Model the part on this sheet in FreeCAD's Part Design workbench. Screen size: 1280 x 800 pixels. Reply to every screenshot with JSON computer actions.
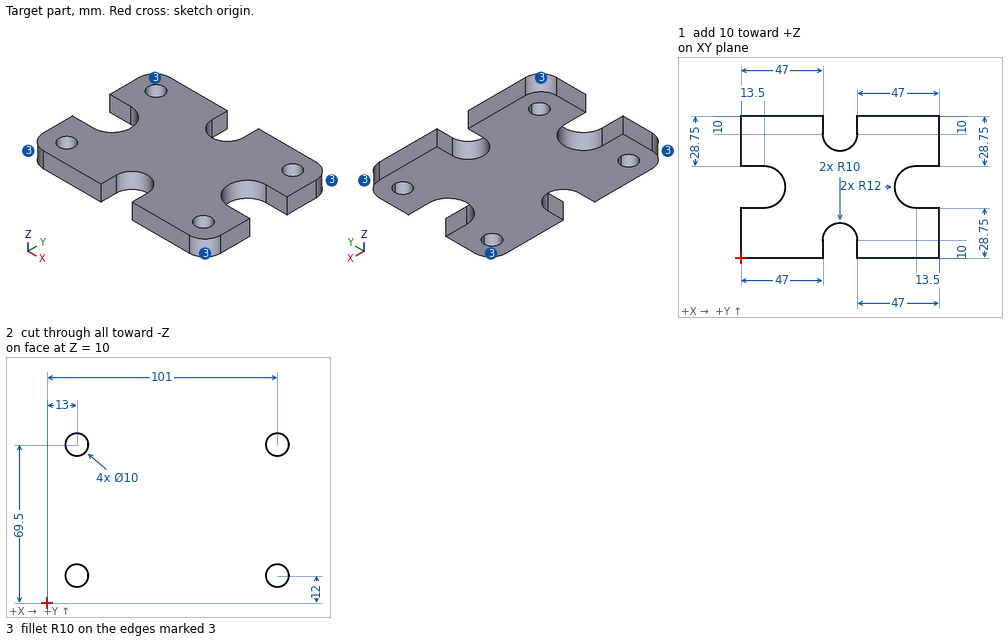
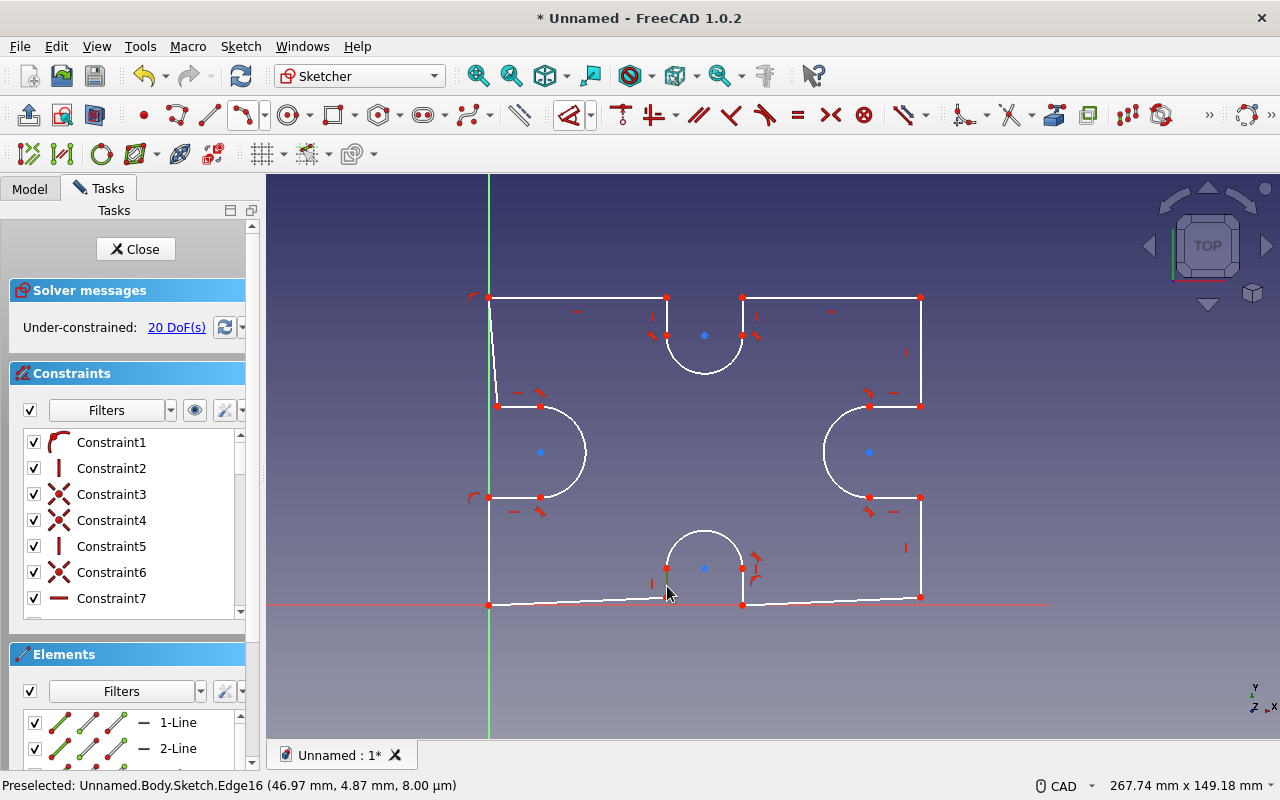
{"action": "left_click", "coordinate": [727, 538]}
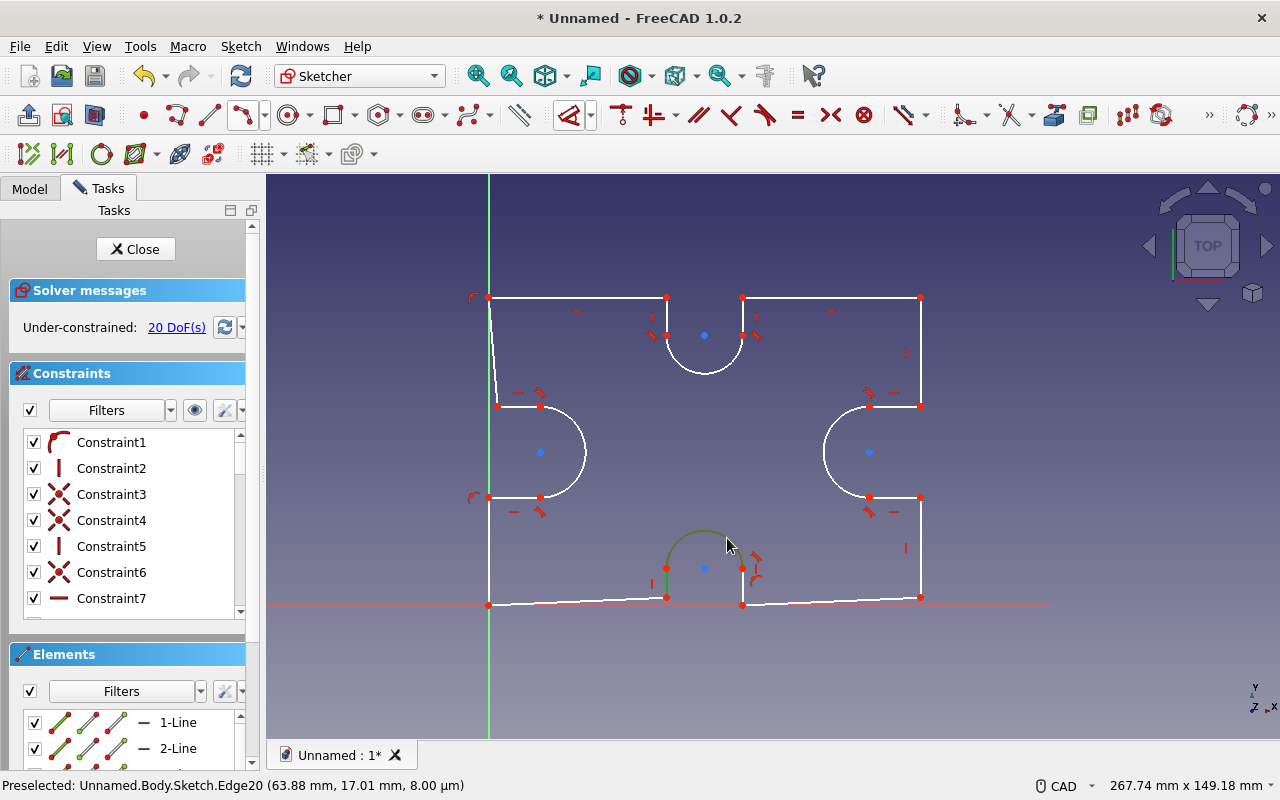
{"action": "left_click", "coordinate": [765, 116]}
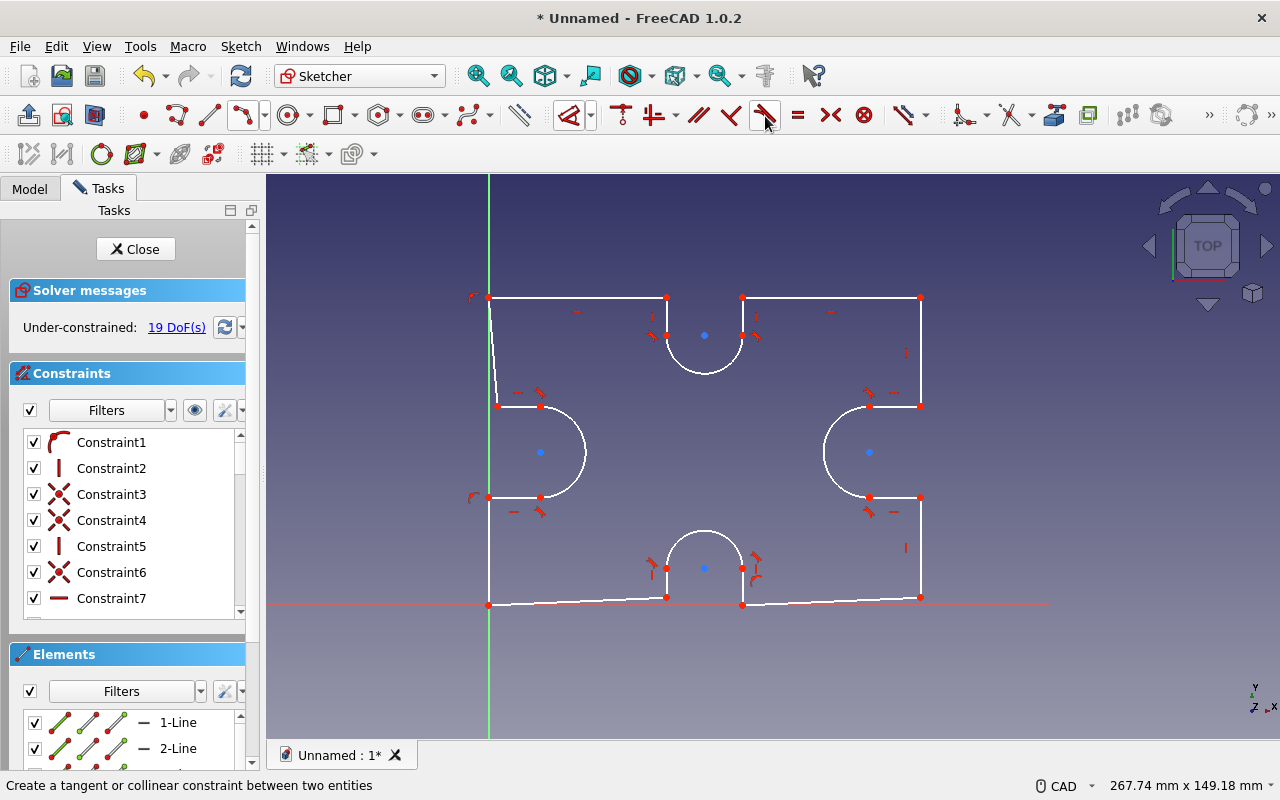
{"action": "left_click", "coordinate": [796, 603]}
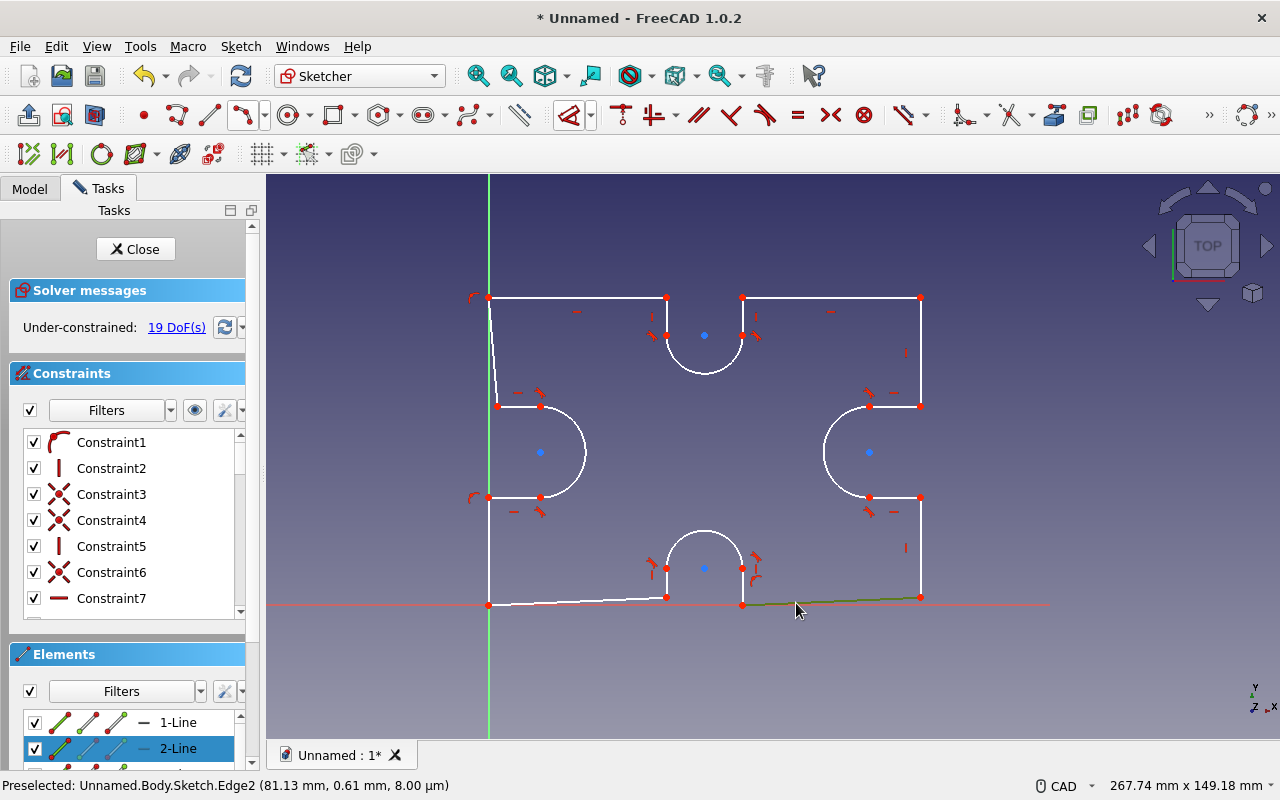
{"action": "left_click", "coordinate": [676, 116]}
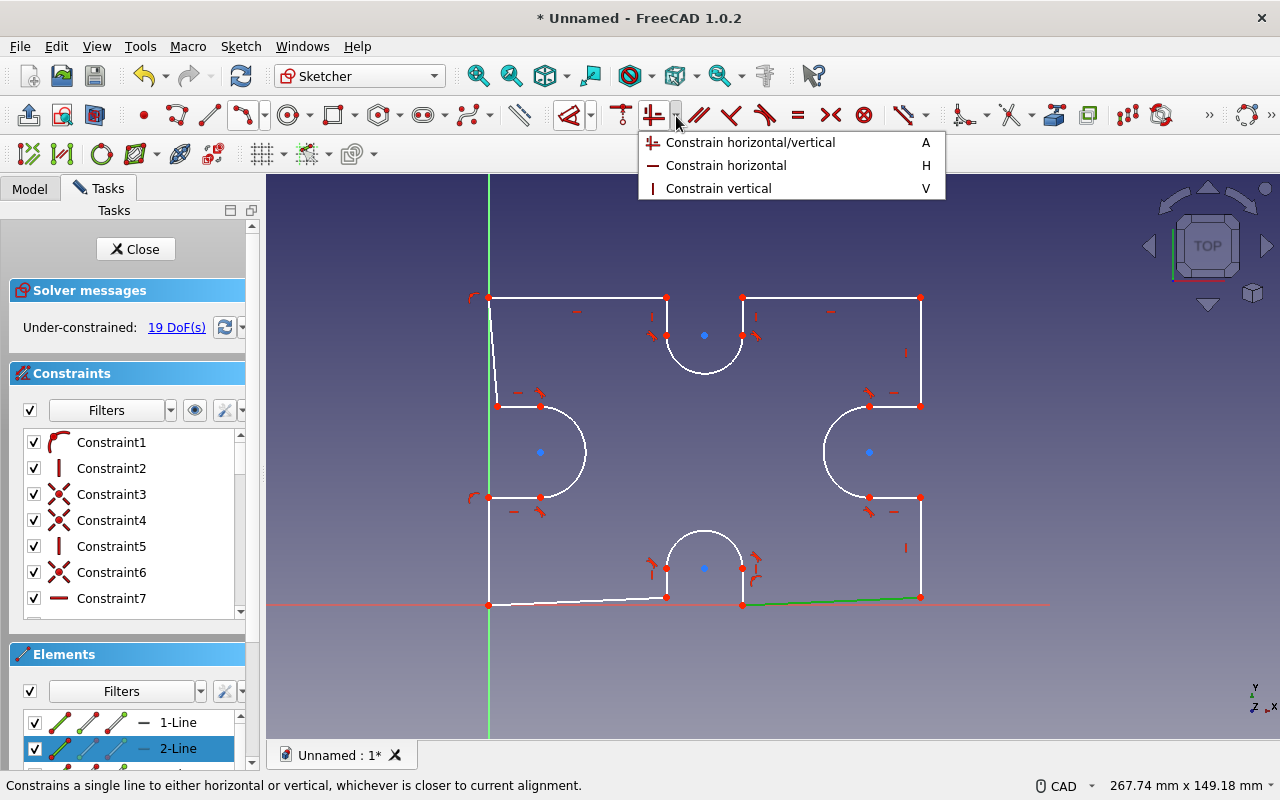
{"action": "left_click", "coordinate": [792, 166]}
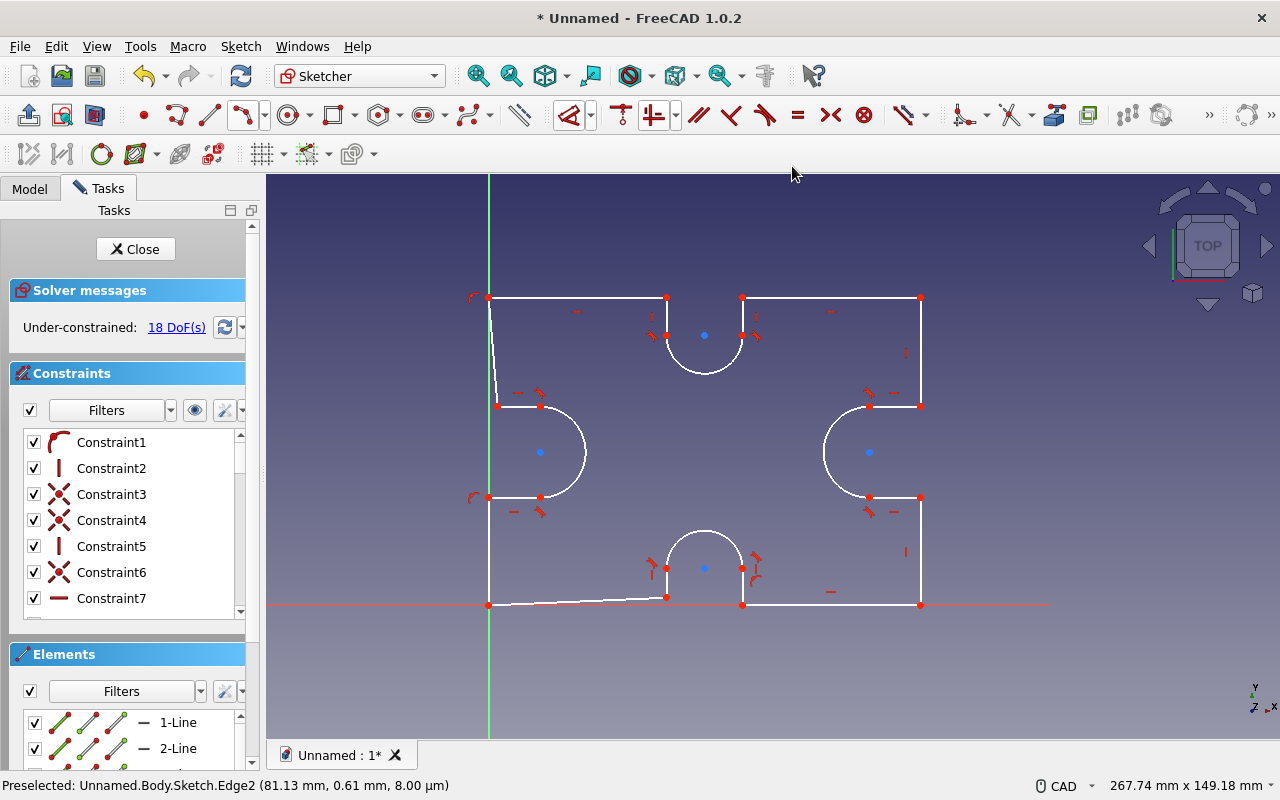
{"action": "left_click", "coordinate": [491, 330]}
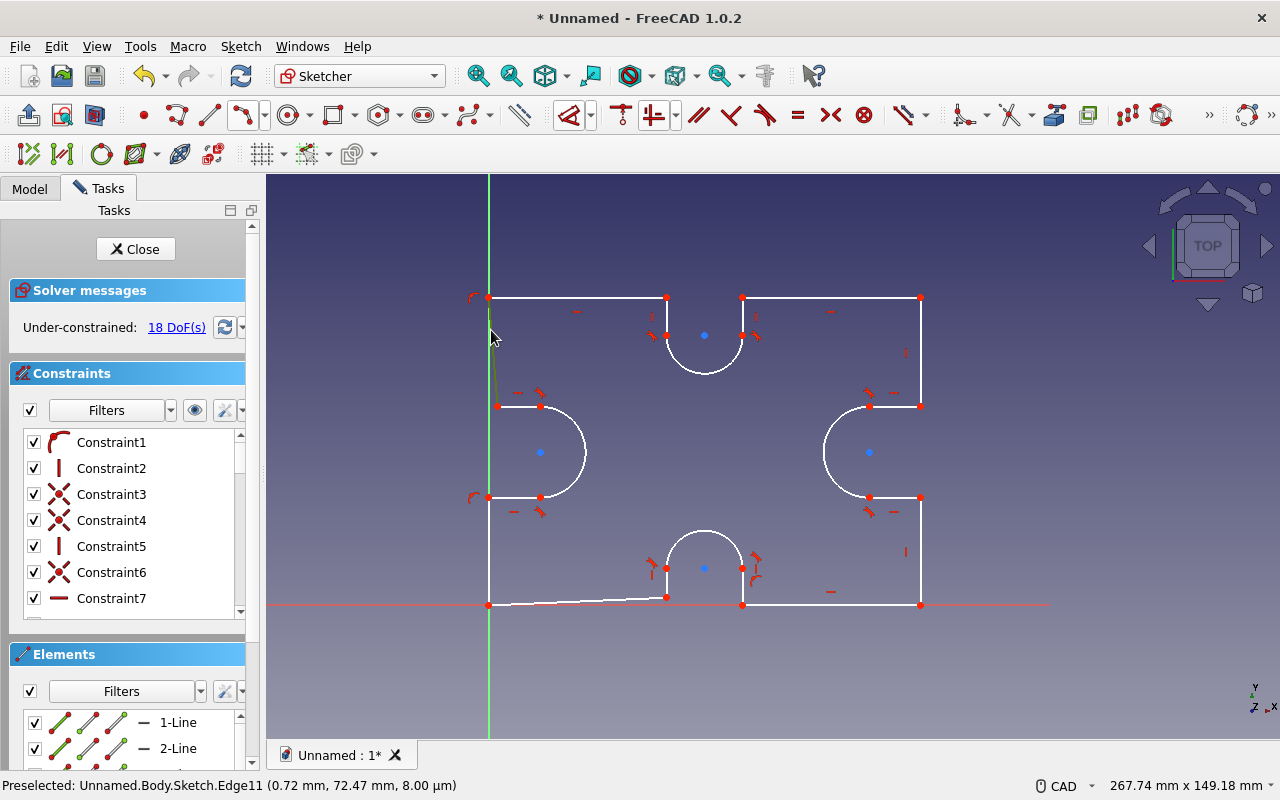
{"action": "key", "text": "v"}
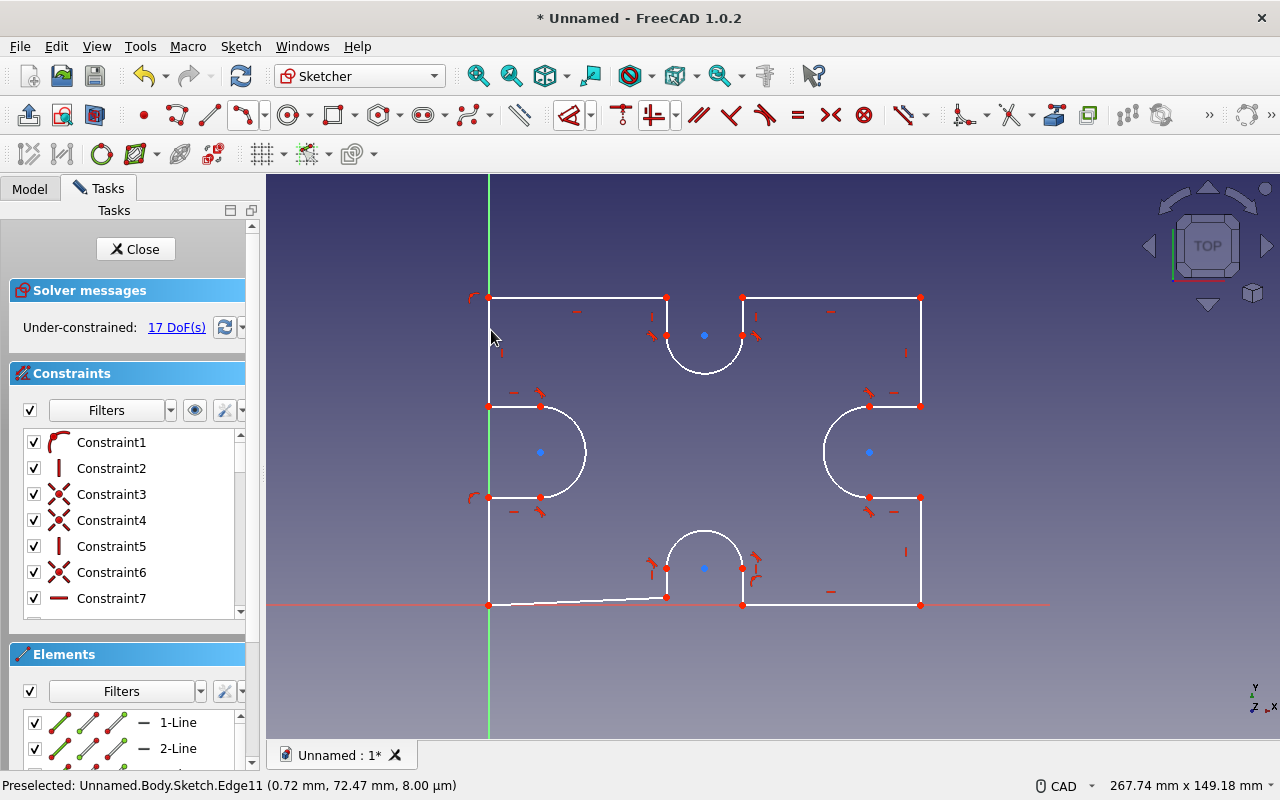
{"action": "left_click", "coordinate": [542, 603]}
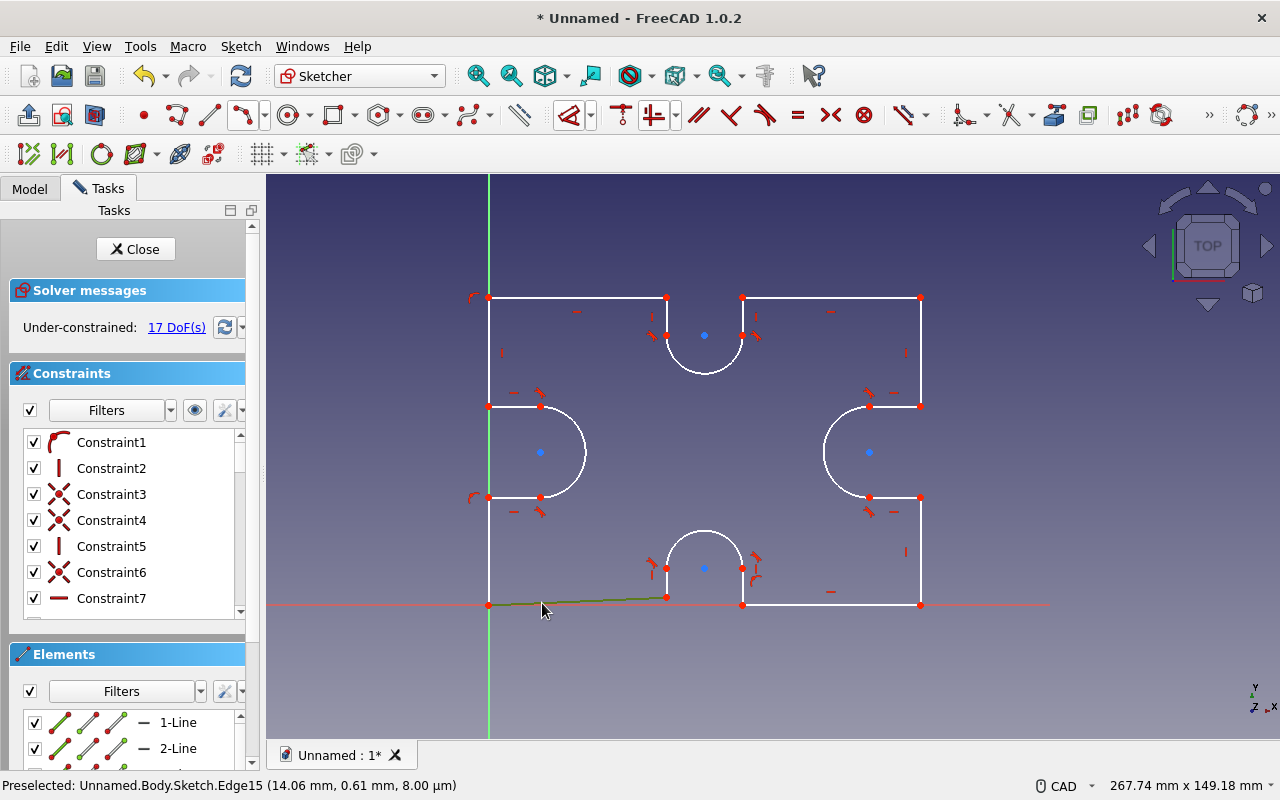
{"action": "key", "text": "h"}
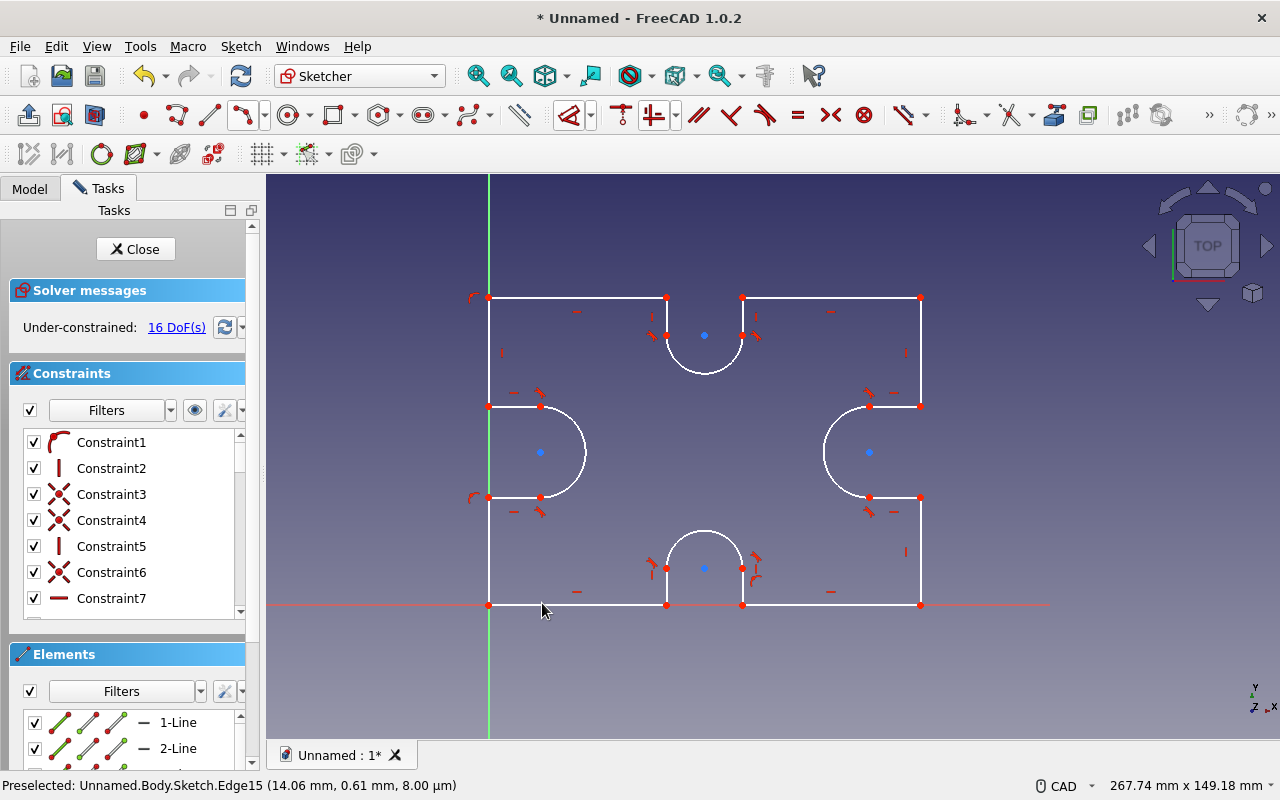
{"action": "left_click", "coordinate": [832, 425]}